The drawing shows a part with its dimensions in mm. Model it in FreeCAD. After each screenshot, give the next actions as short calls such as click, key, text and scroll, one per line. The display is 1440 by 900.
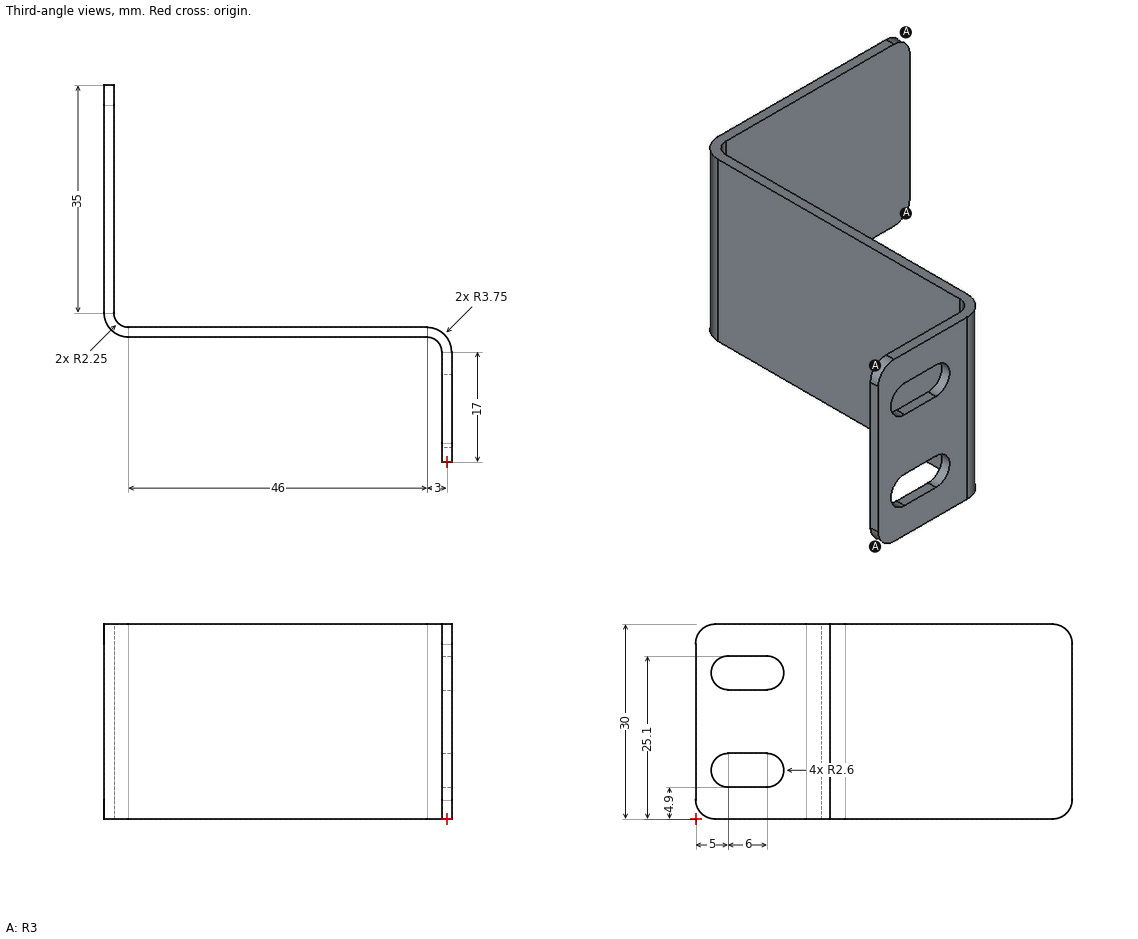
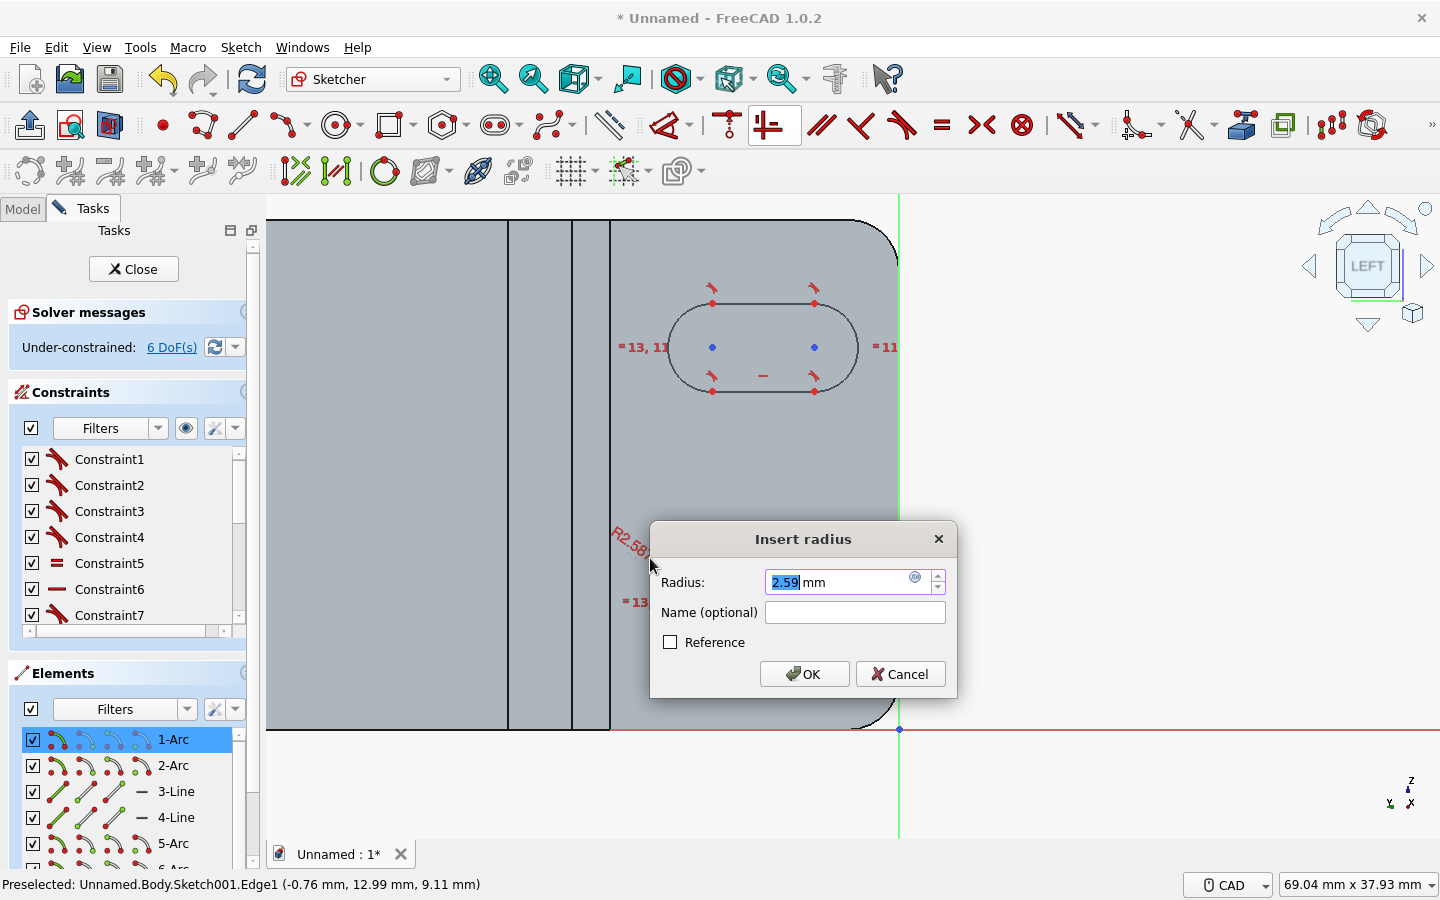
text(2.6)
key(Return)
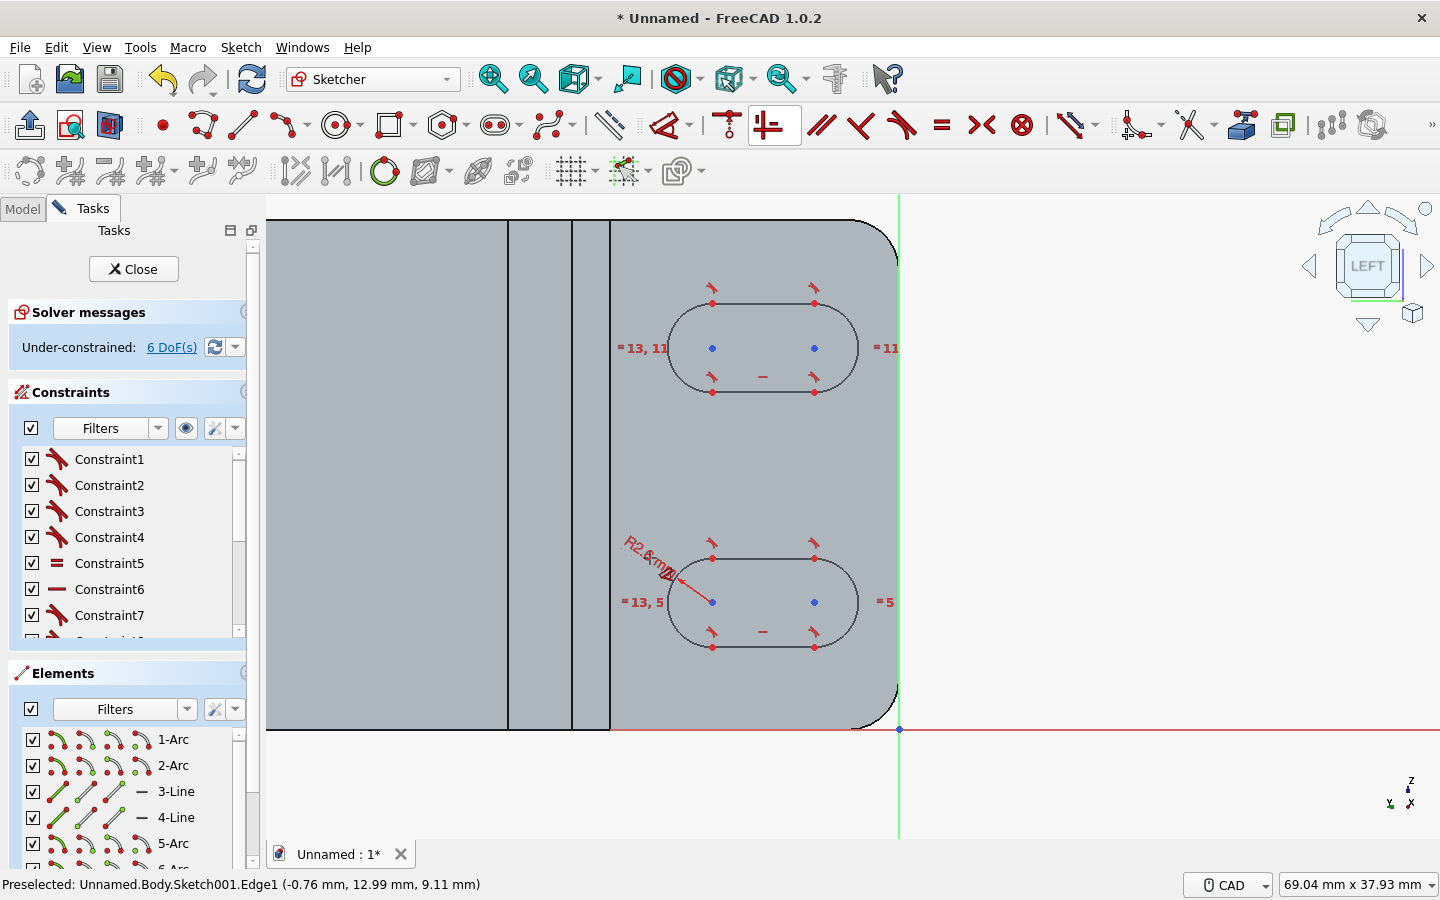
click(743, 559)
click(763, 593)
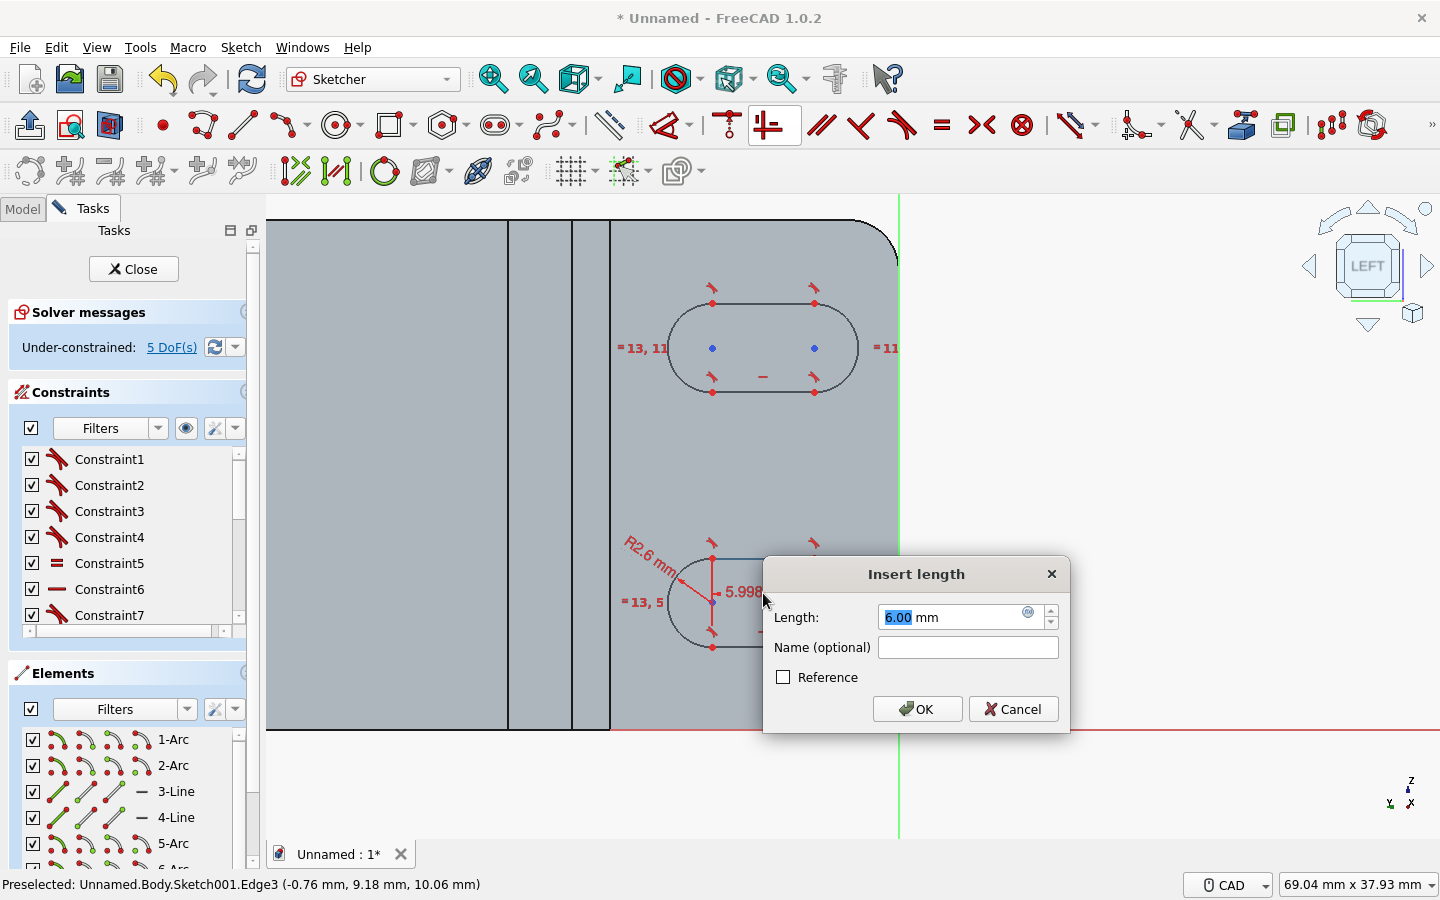
text(6)
key(Return)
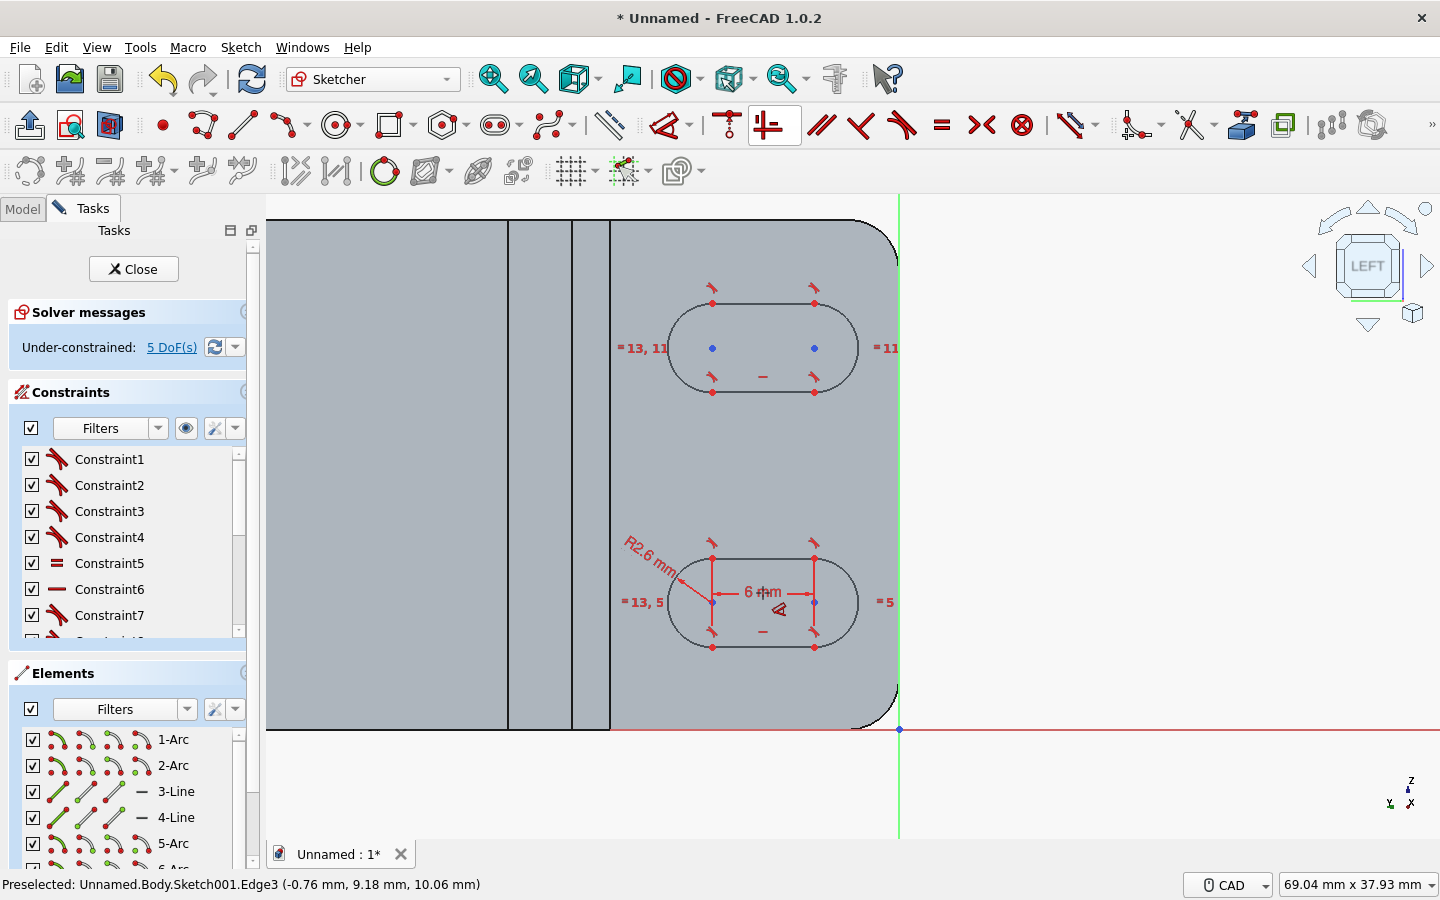
click(743, 304)
click(763, 270)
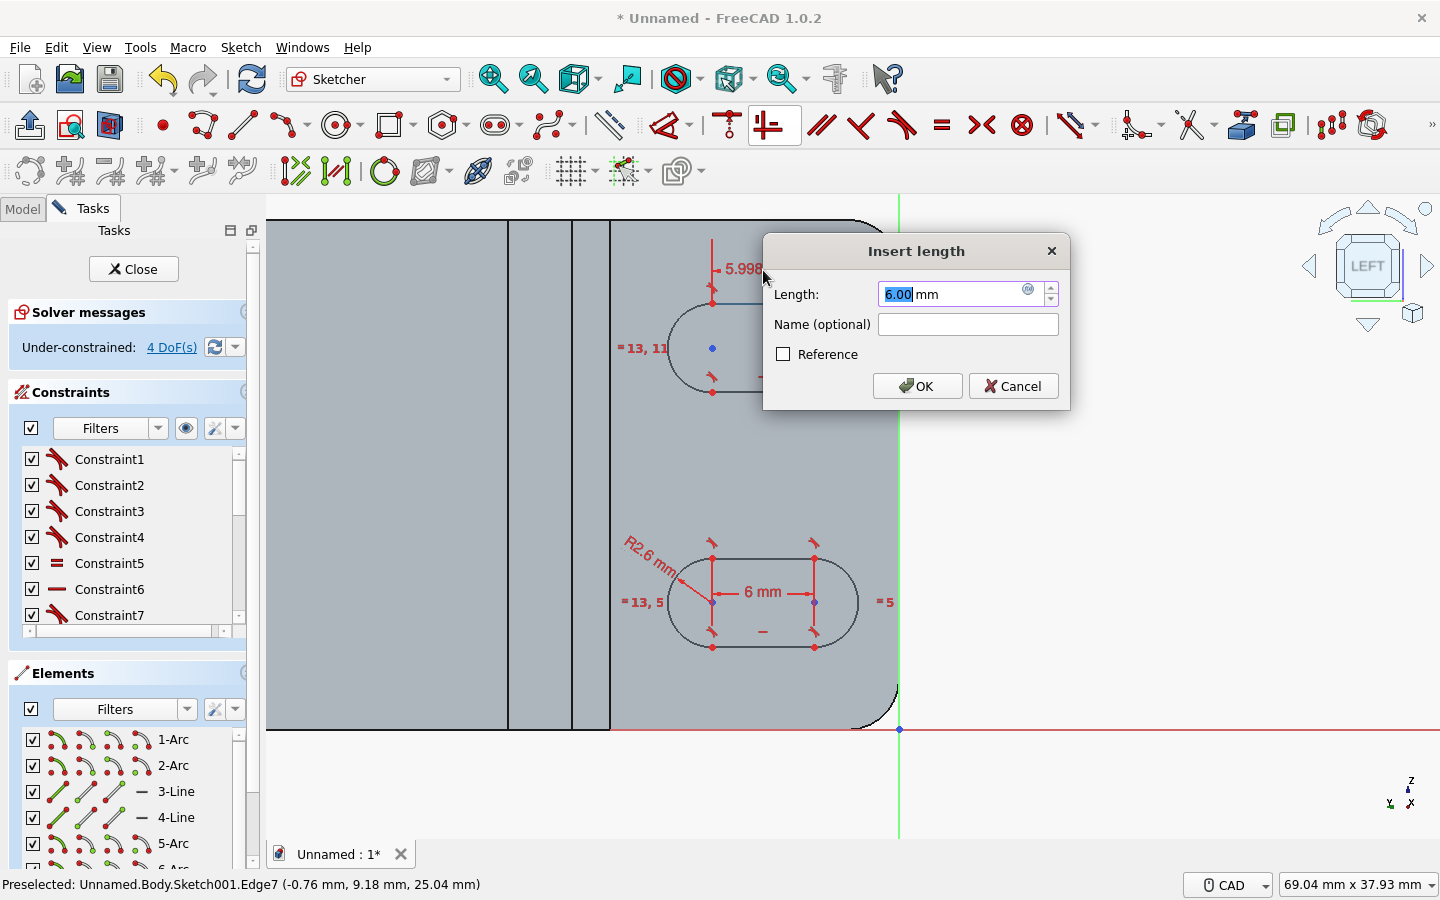
text(6)
key(Return)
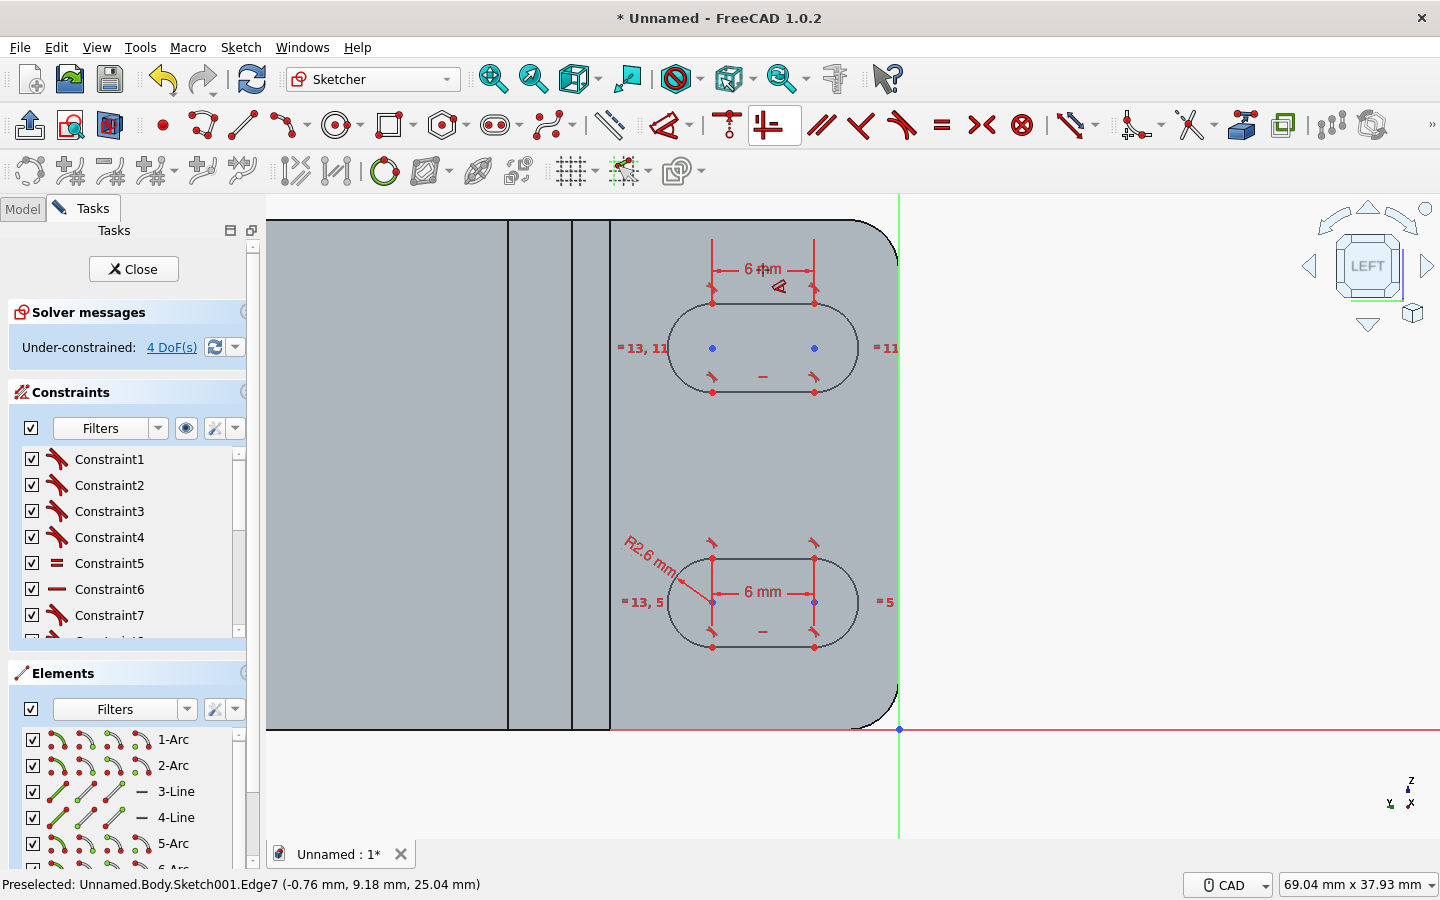
click(814, 647)
click(857, 764)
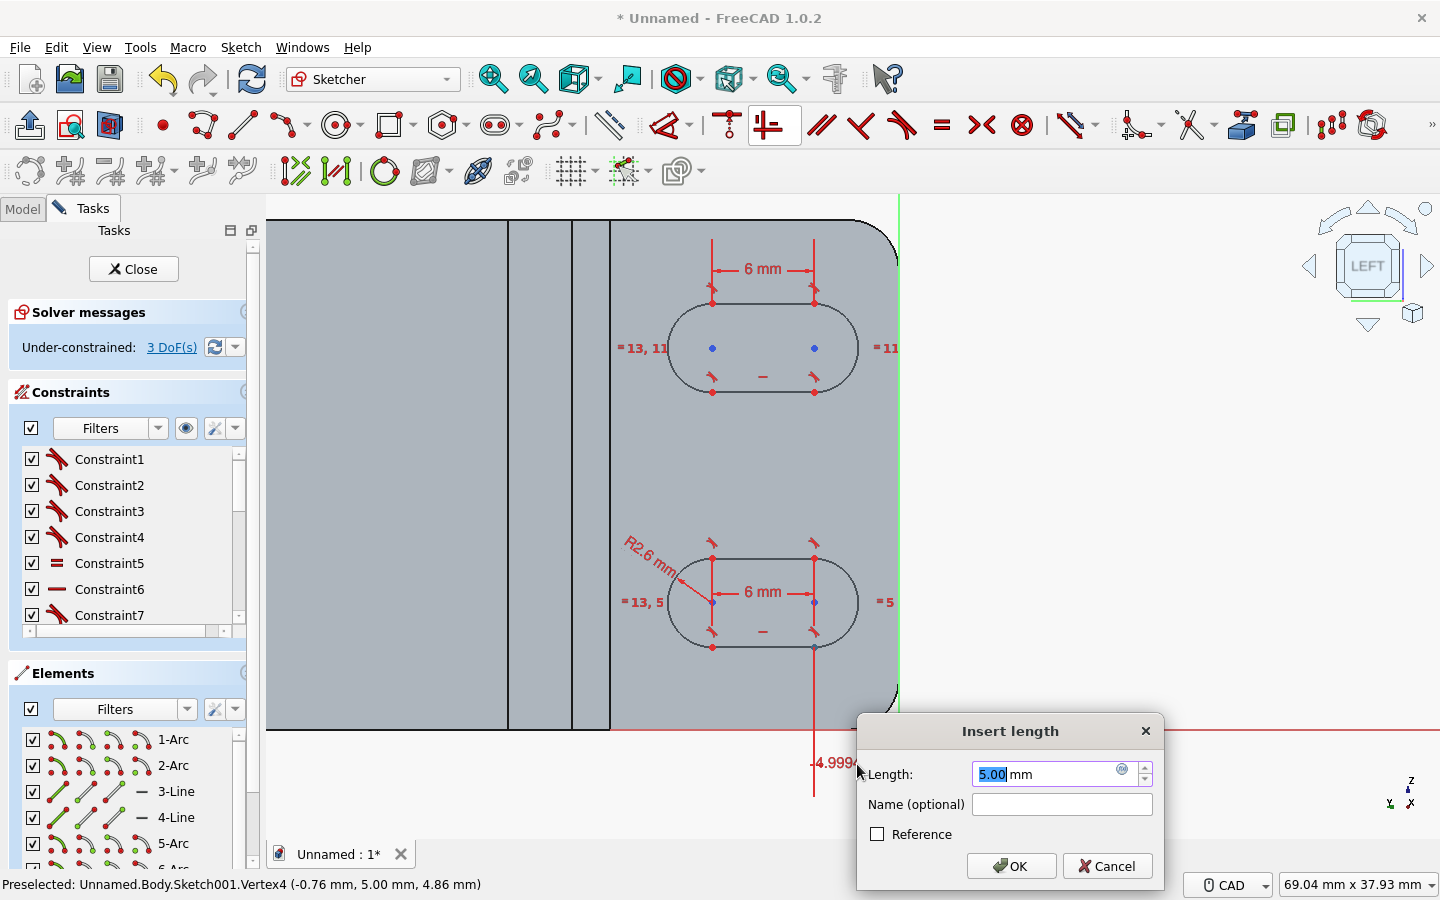
text(5)
key(Return)